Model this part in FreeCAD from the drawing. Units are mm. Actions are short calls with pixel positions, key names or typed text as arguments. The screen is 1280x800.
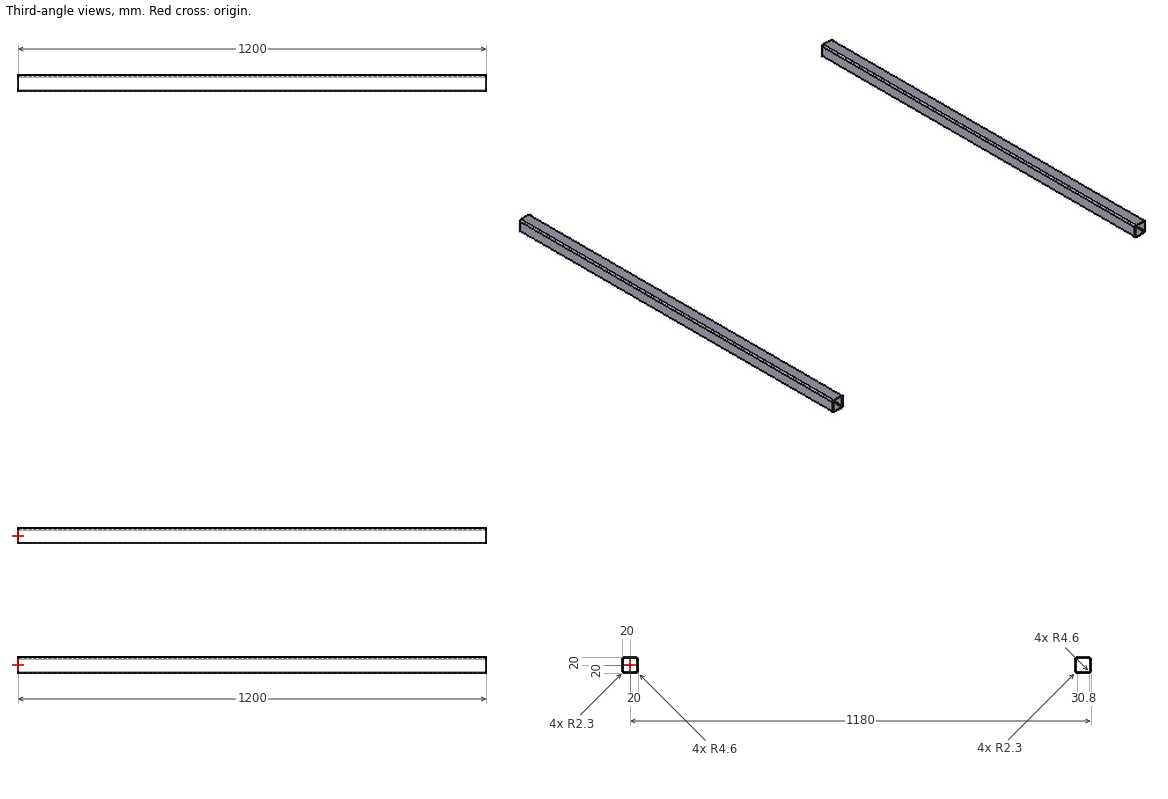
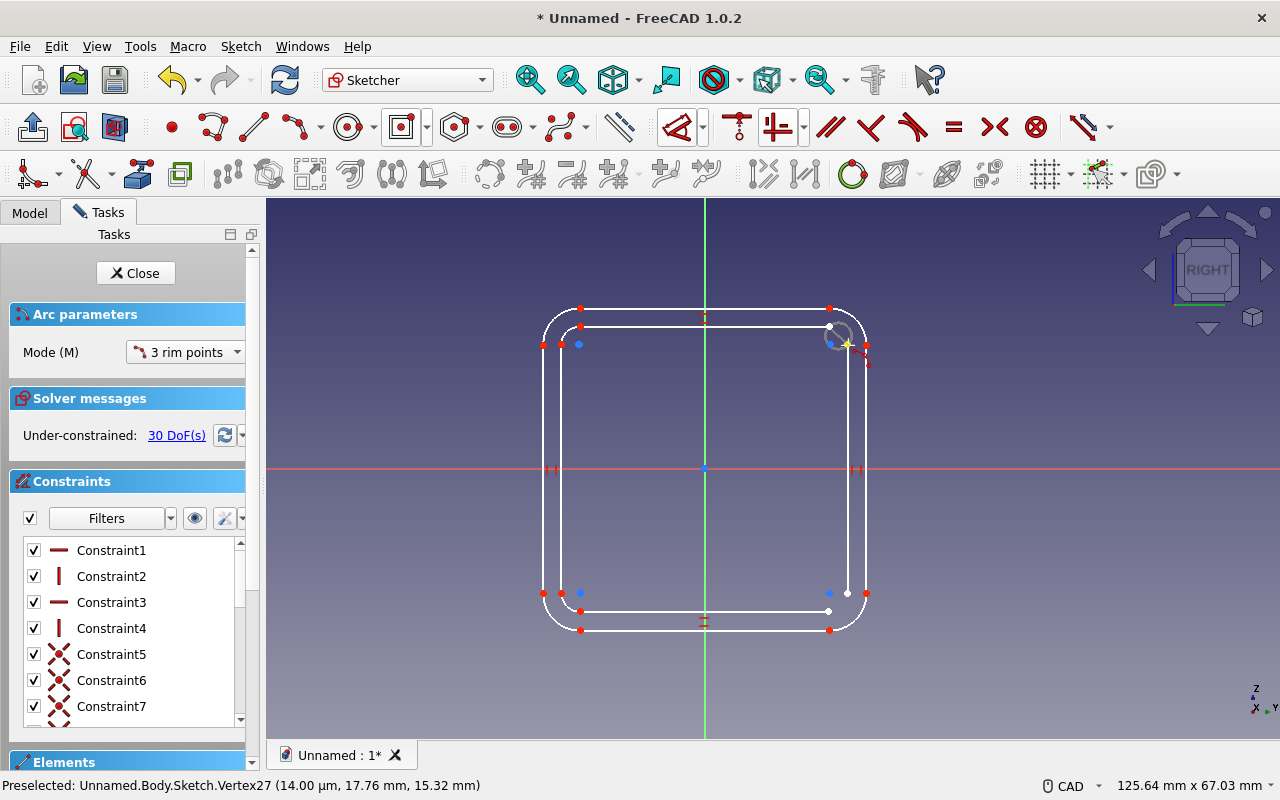
scroll(842, 331, up, 6)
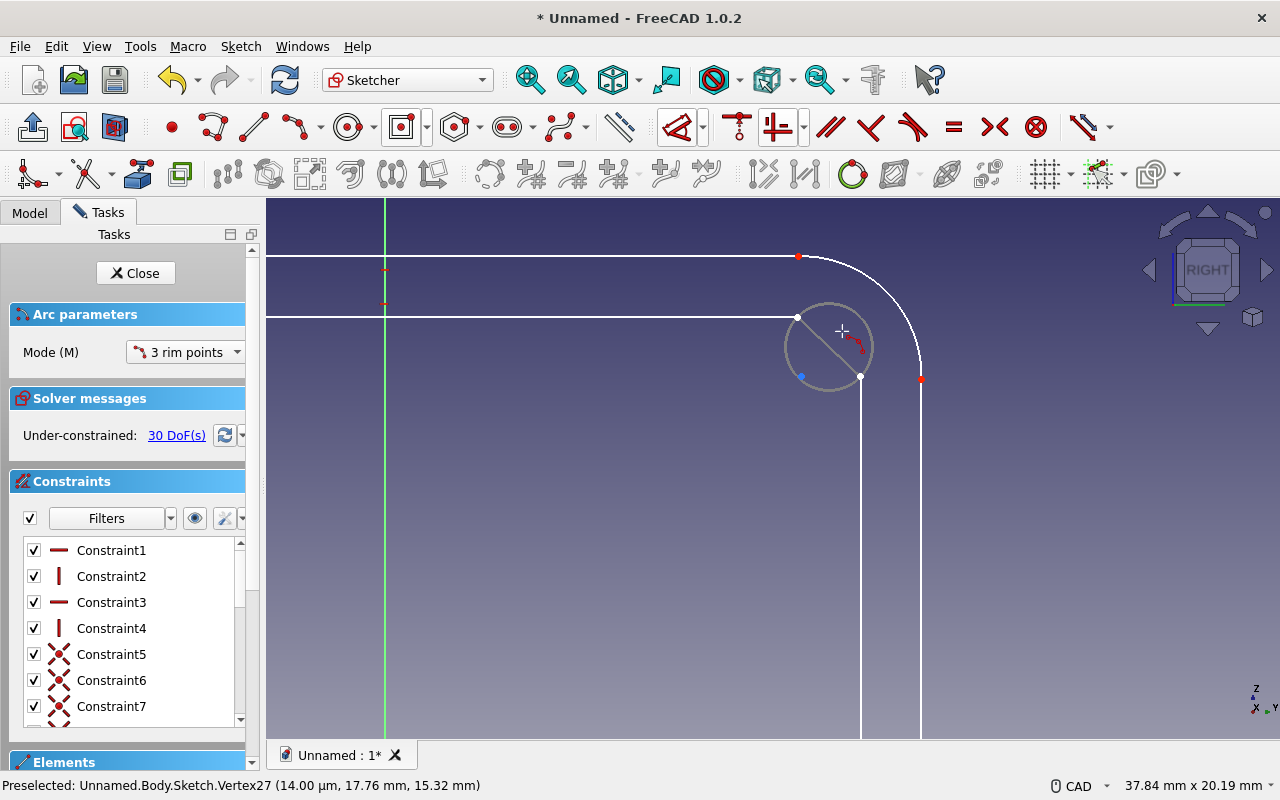
click(841, 331)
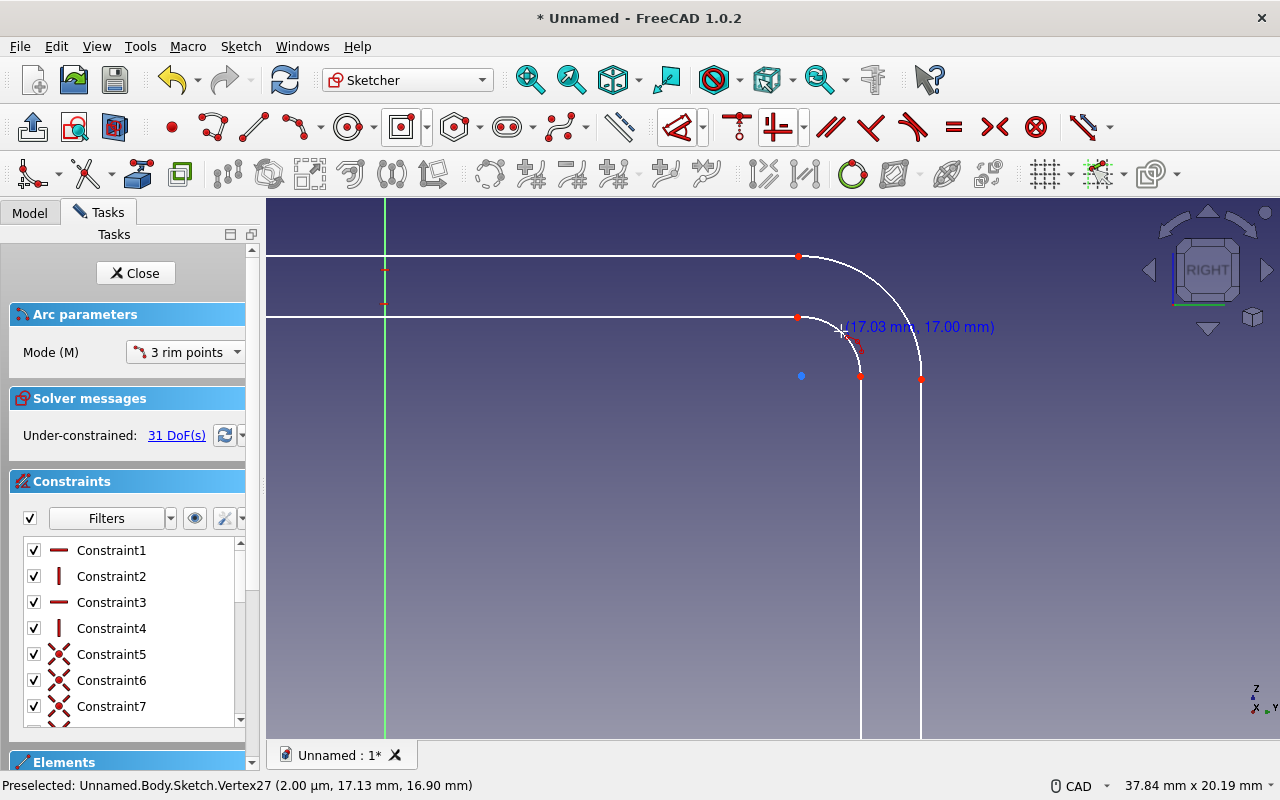
scroll(842, 331, down, 6)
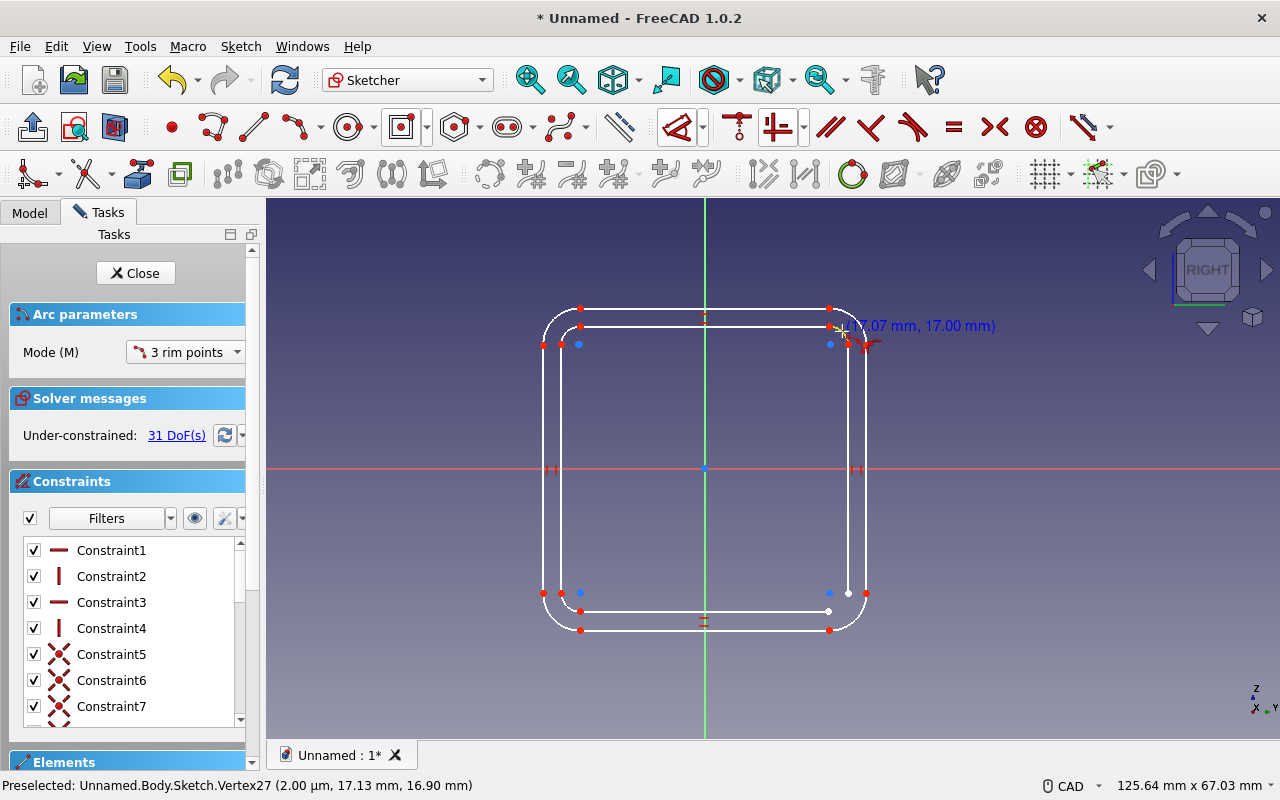
click(848, 594)
click(829, 612)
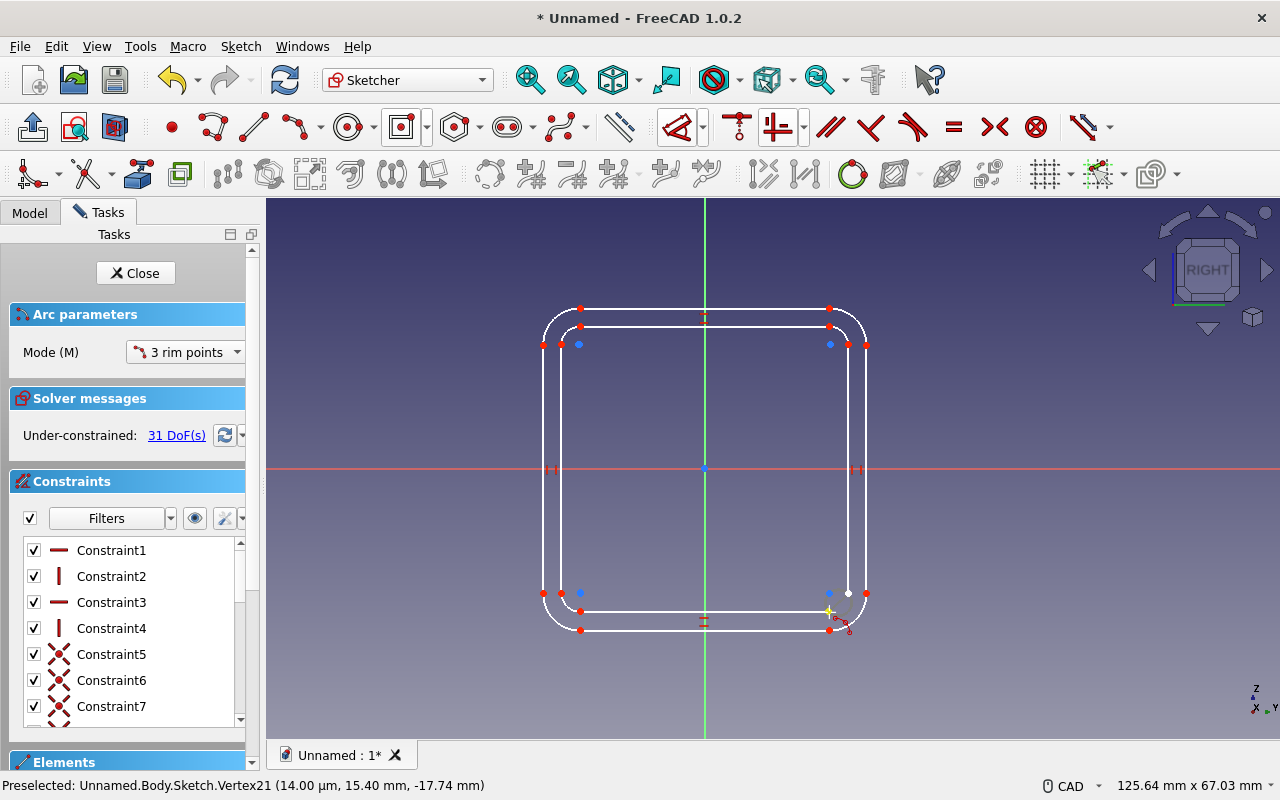
scroll(842, 606, up, 6)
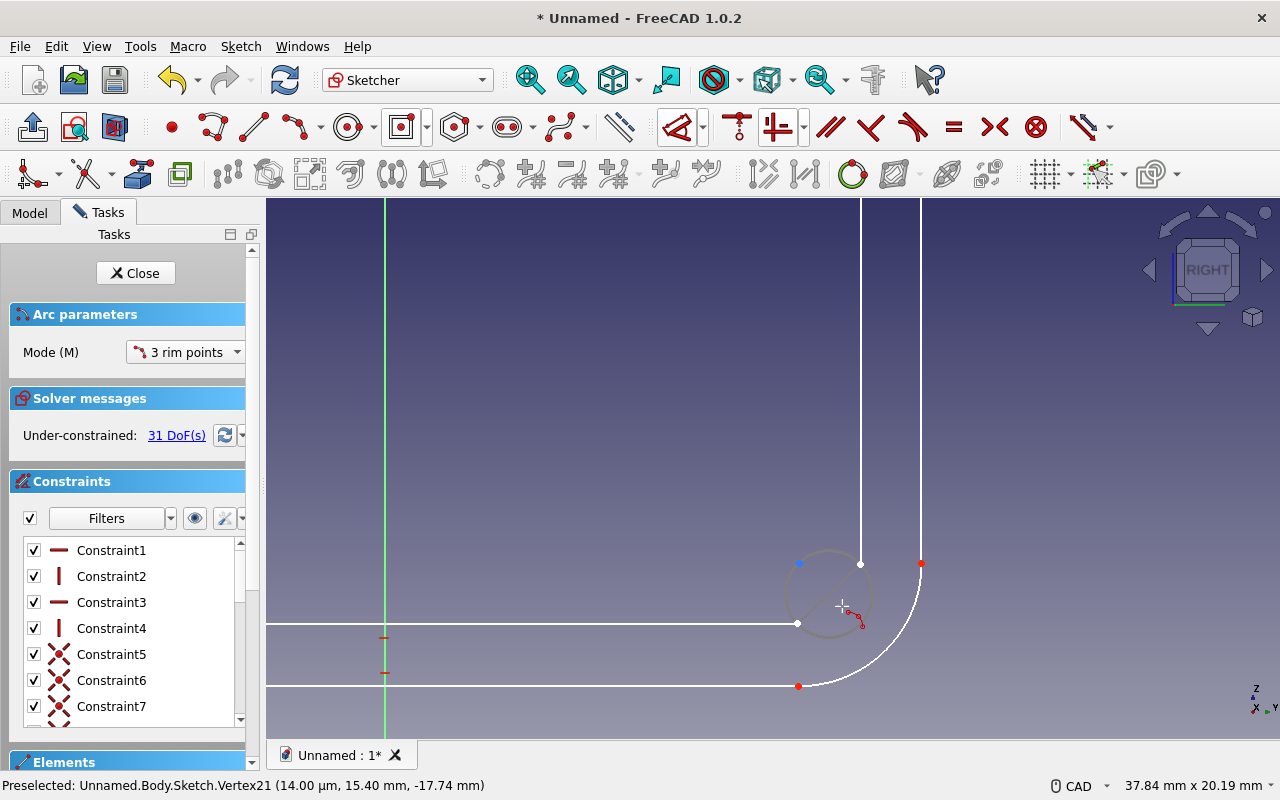
click(841, 605)
key(Escape)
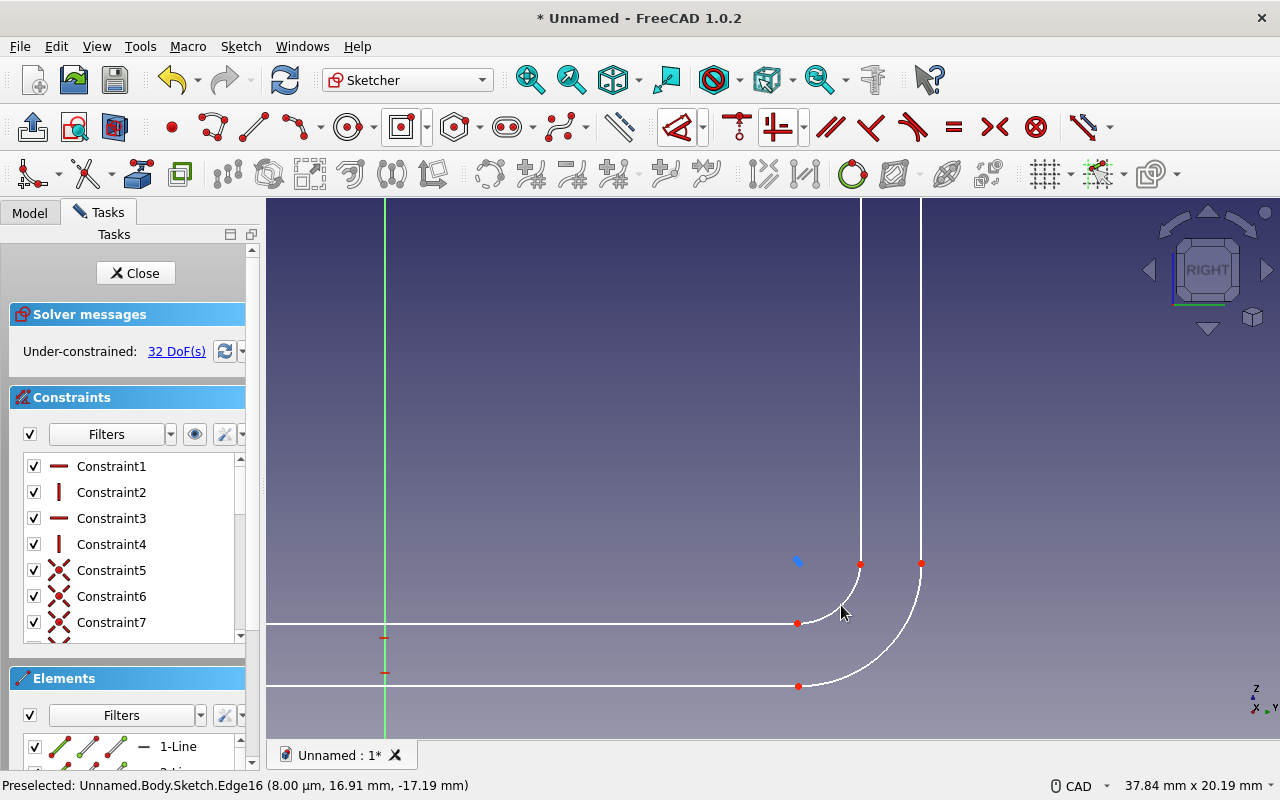
click(551, 686)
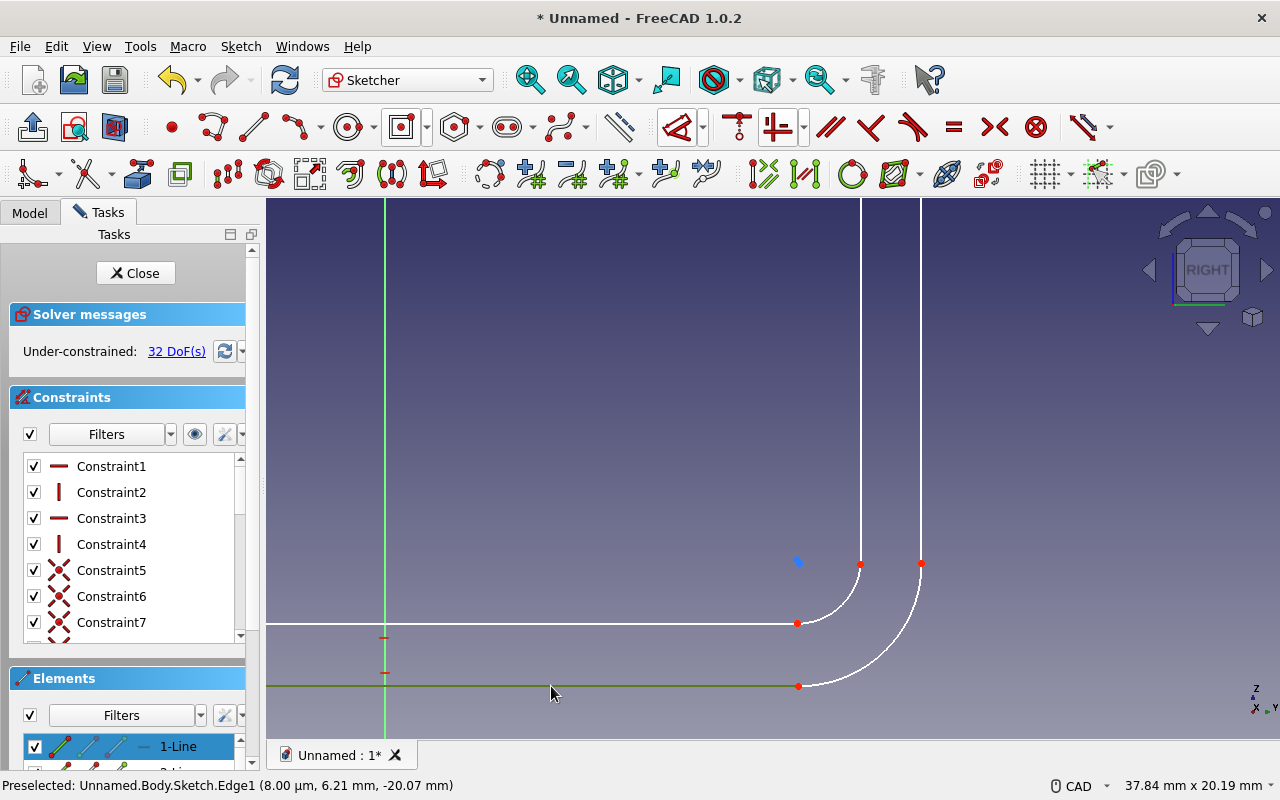
click(855, 673)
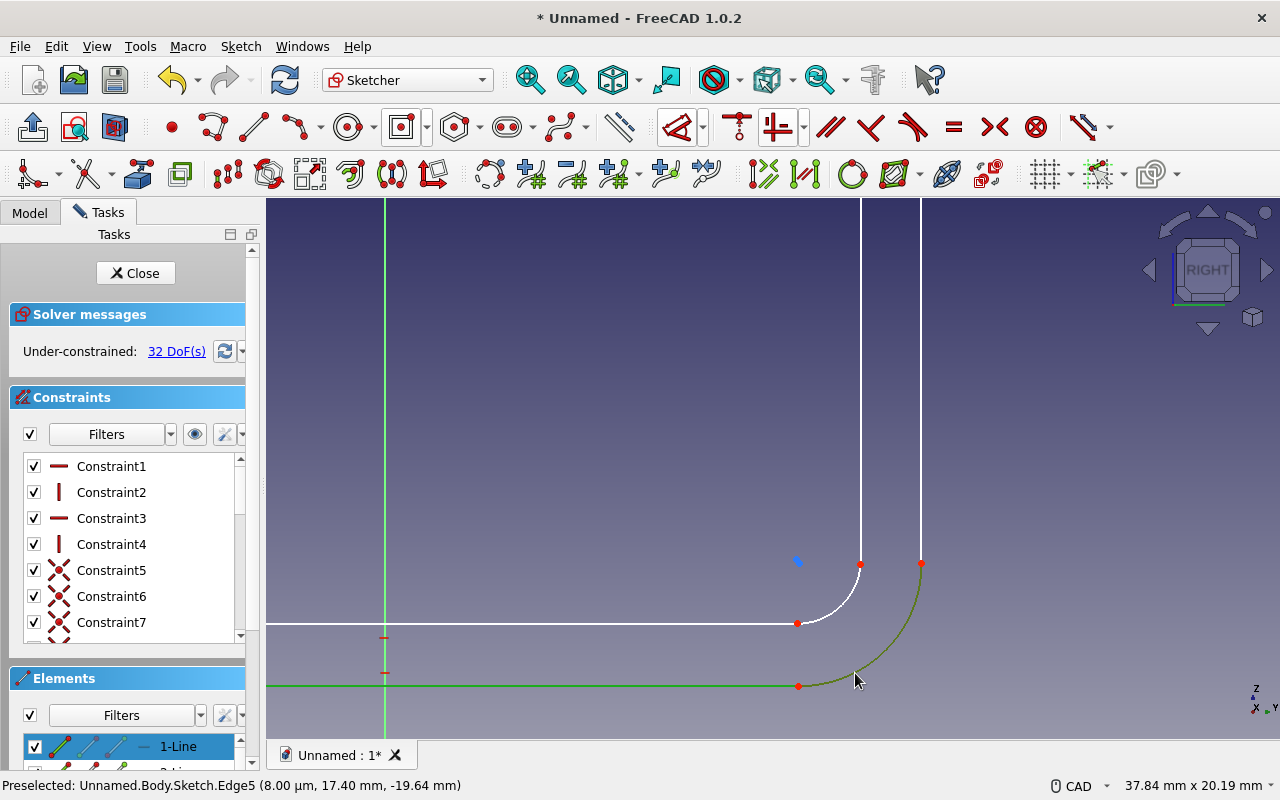
key(t)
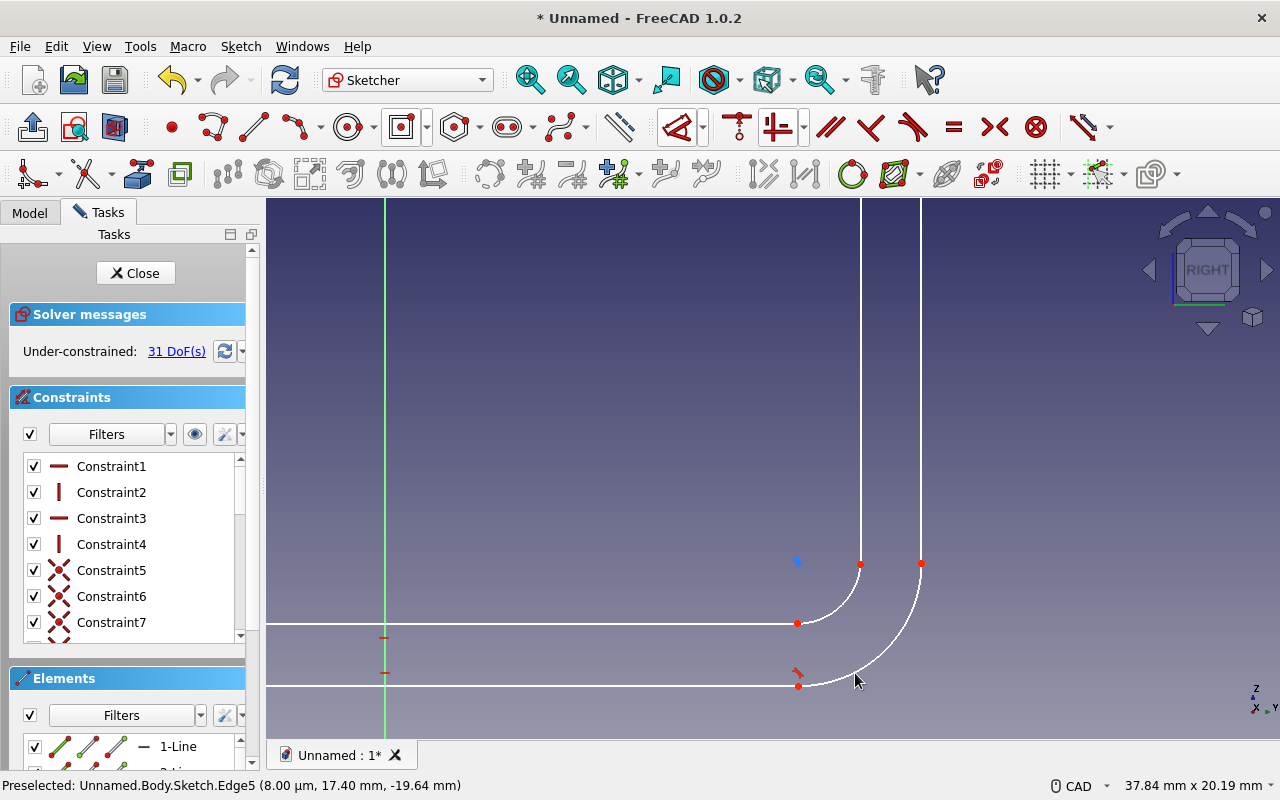
click(551, 686)